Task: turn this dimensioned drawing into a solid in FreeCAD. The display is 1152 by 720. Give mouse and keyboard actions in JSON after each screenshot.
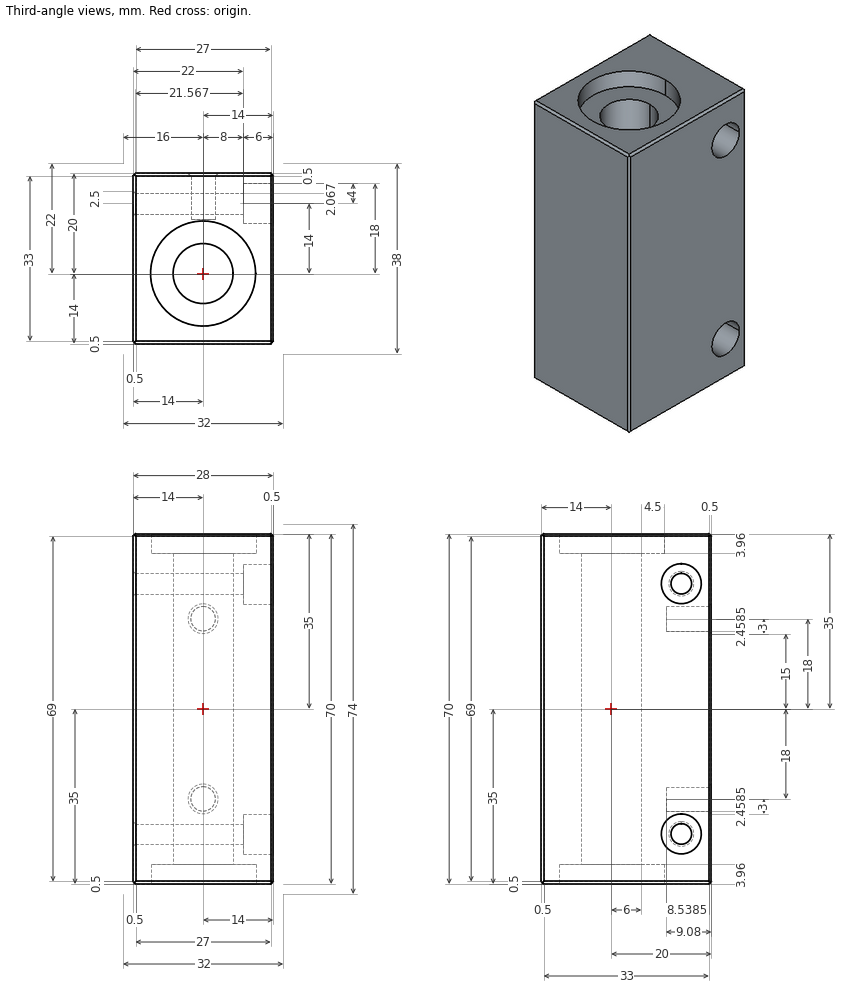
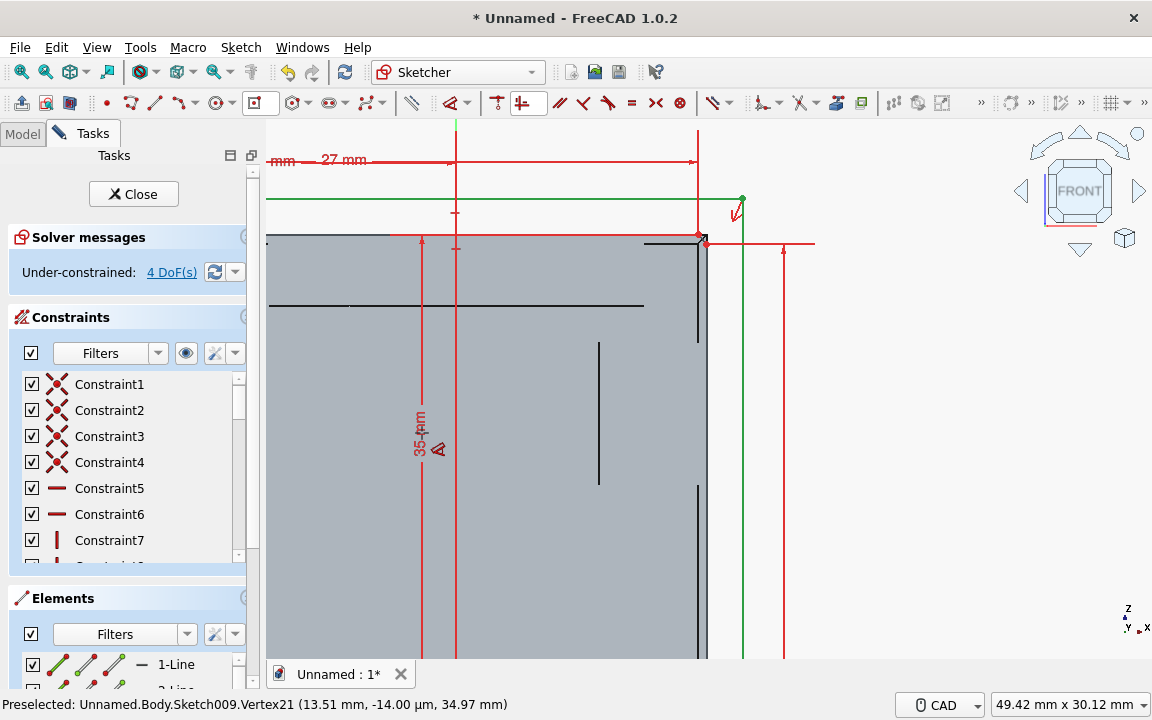
{"action": "scroll", "coordinate": [701, 234], "scroll_direction": "down", "scroll_amount": 7}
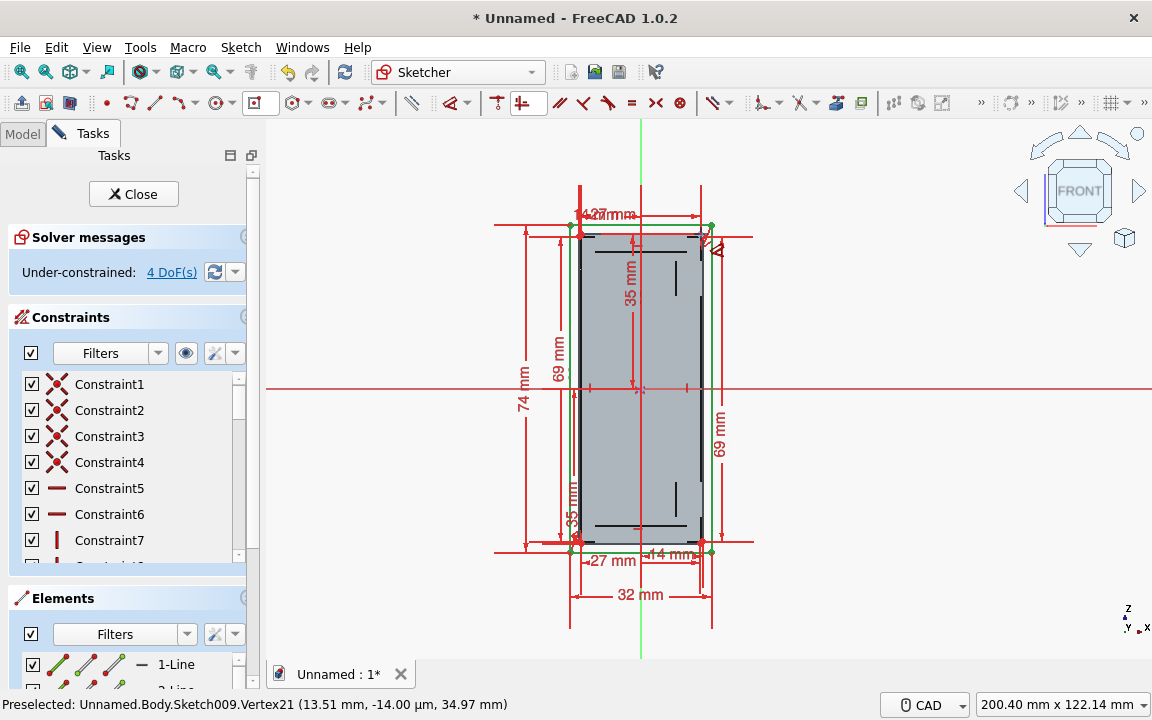
{"action": "scroll", "coordinate": [580, 543], "scroll_direction": "up", "scroll_amount": 15}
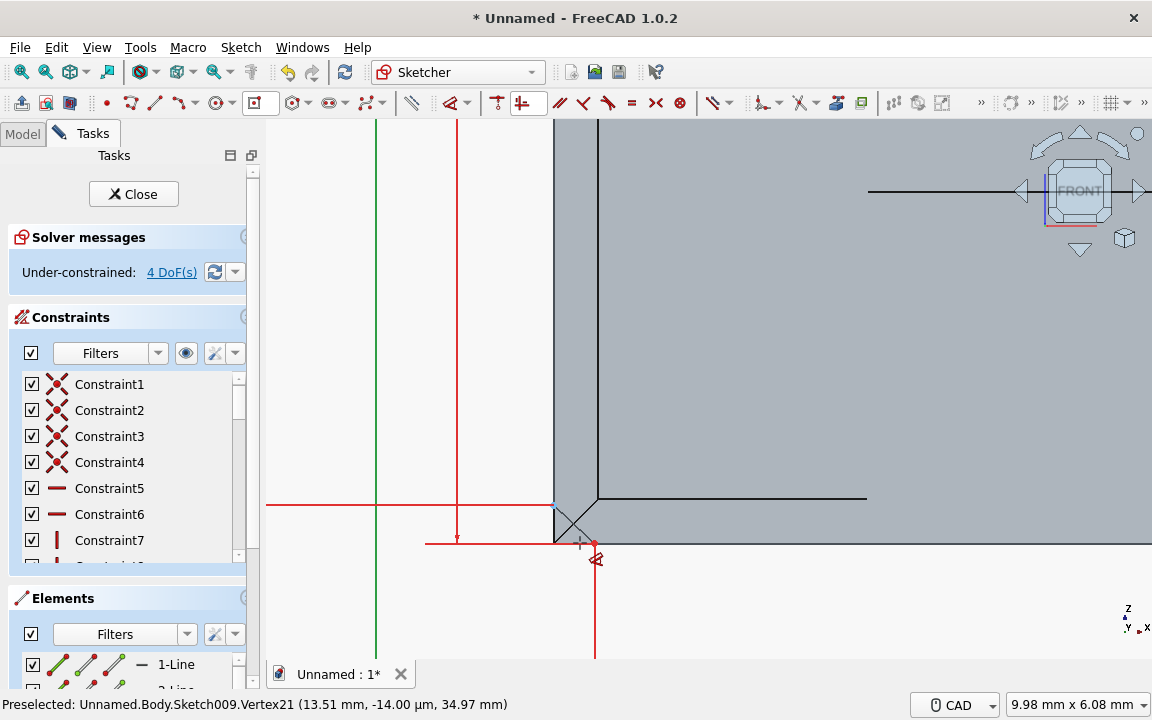
{"action": "left_click", "coordinate": [574, 525]}
{"action": "left_click", "coordinate": [574, 578]}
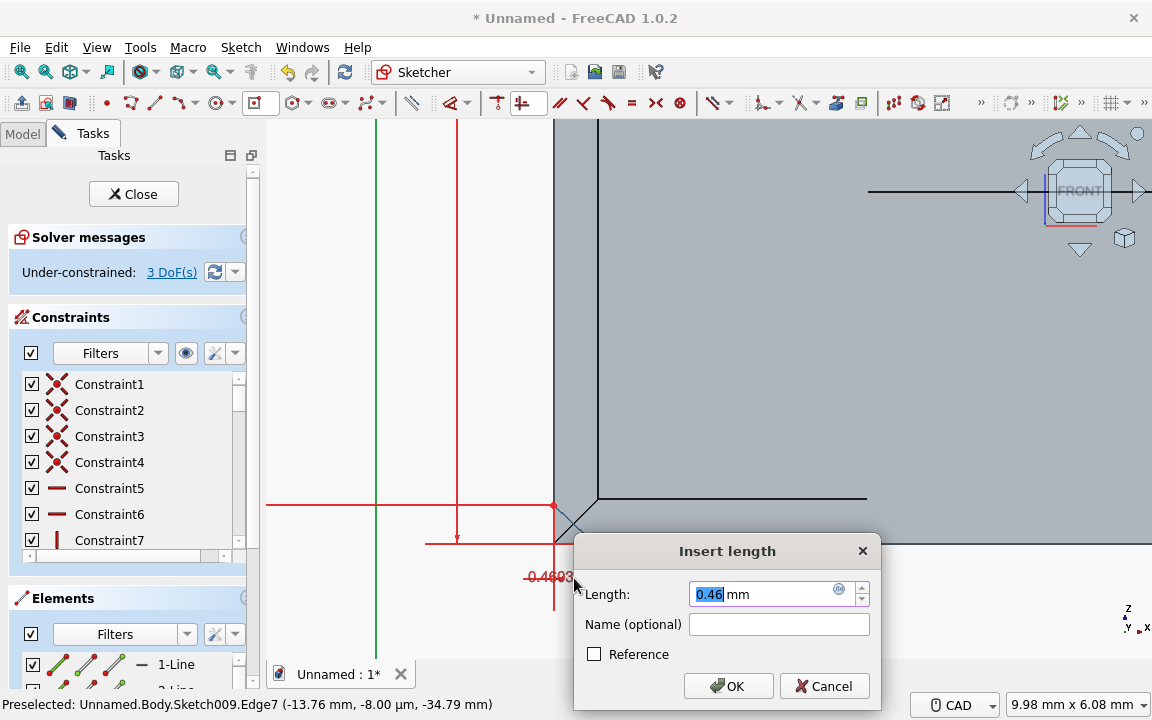
{"action": "type", "text": "0.5"}
{"action": "key", "text": "Return"}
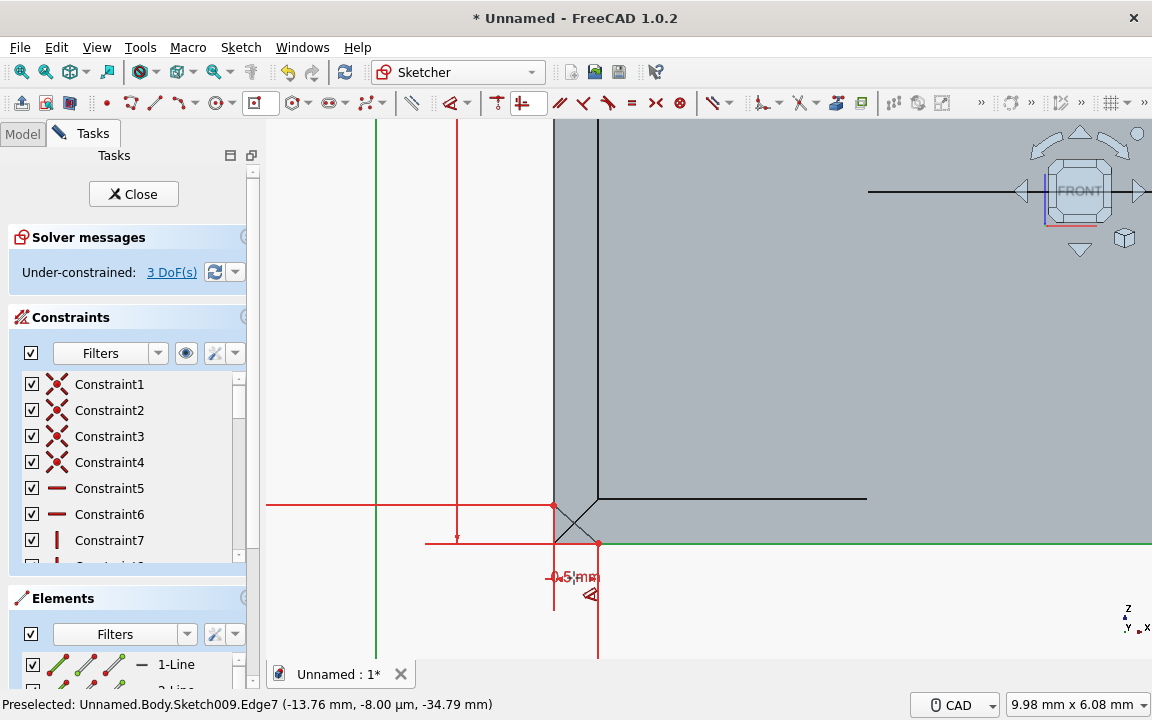
{"action": "left_click", "coordinate": [567, 517]}
{"action": "left_click", "coordinate": [520, 525]}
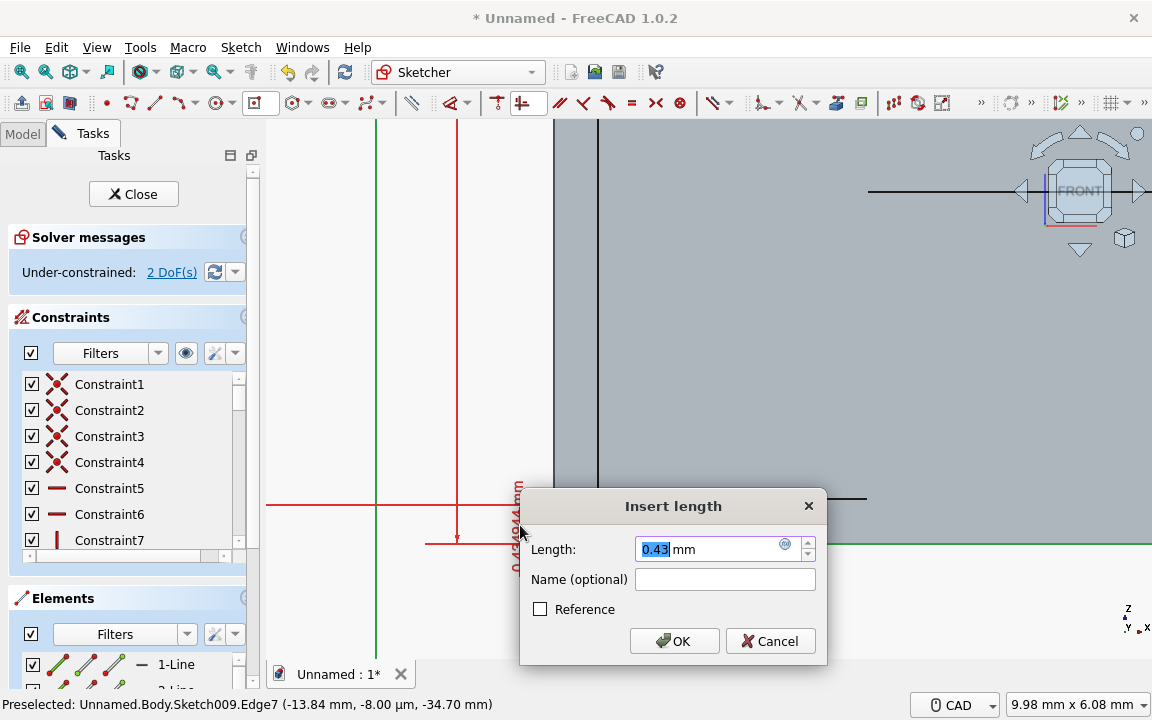
{"action": "type", "text": "0.5"}
{"action": "key", "text": "Return"}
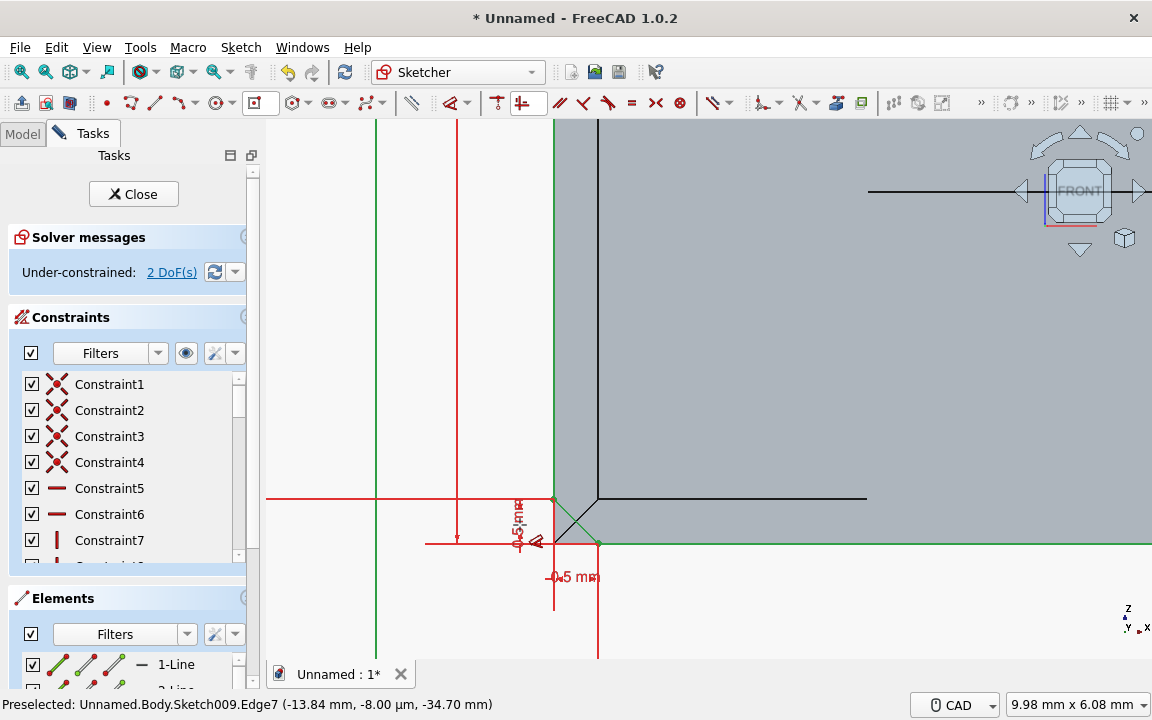
{"action": "scroll", "coordinate": [580, 544], "scroll_direction": "down", "scroll_amount": 15}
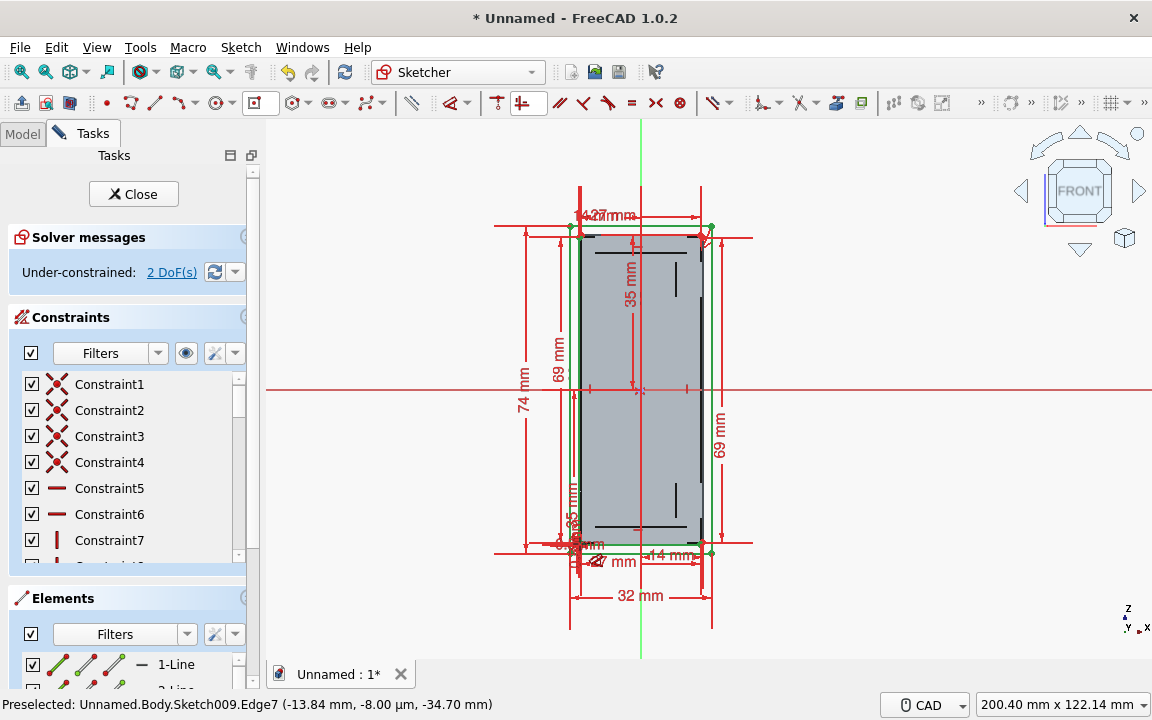
{"action": "scroll", "coordinate": [701, 544], "scroll_direction": "up", "scroll_amount": 15}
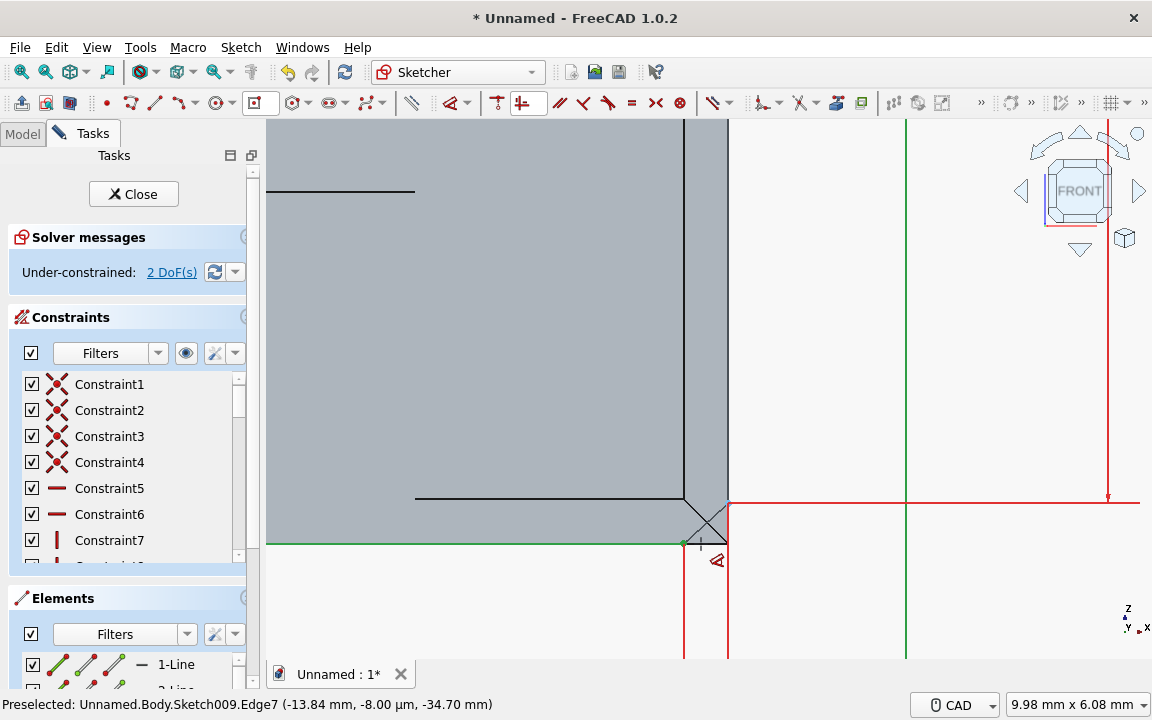
{"action": "left_click", "coordinate": [697, 532]}
{"action": "left_click", "coordinate": [762, 524]}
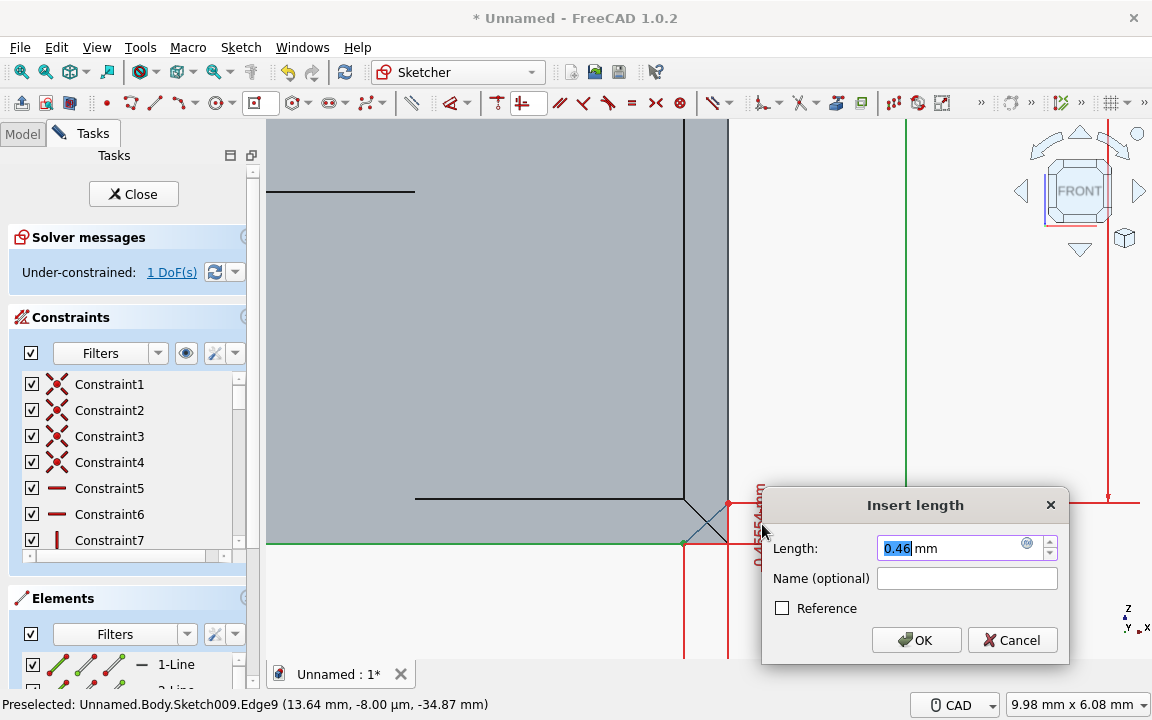
{"action": "type", "text": "0.5"}
{"action": "key", "text": "Return"}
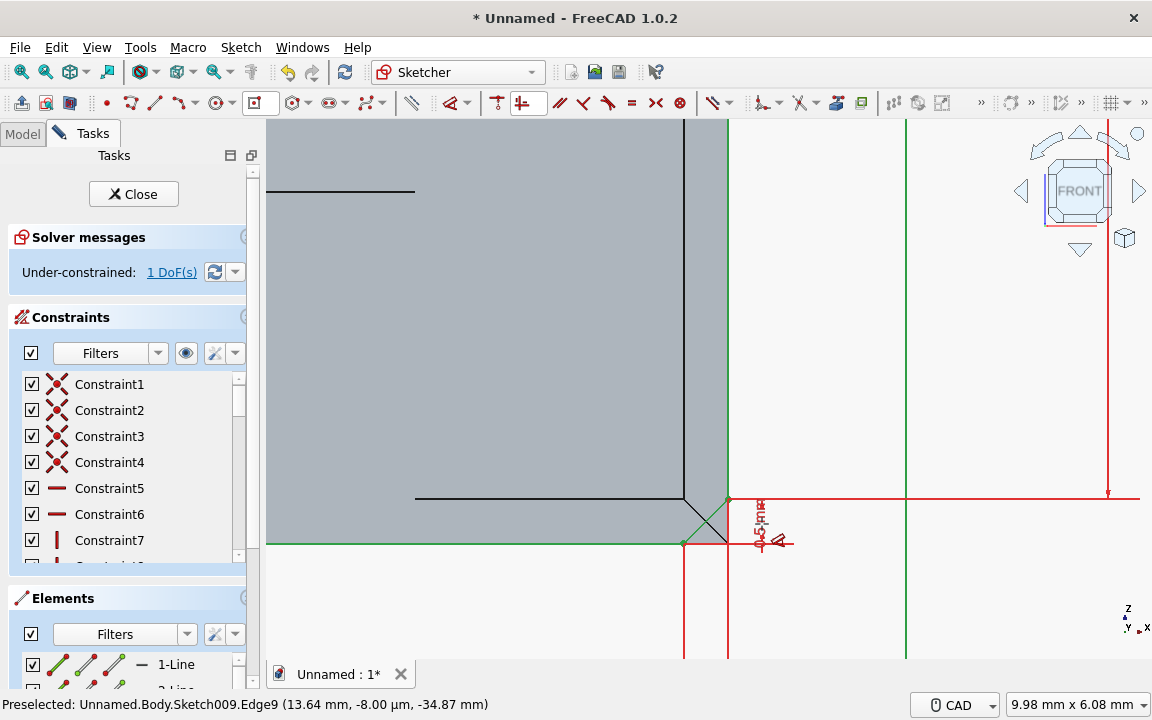
{"action": "scroll", "coordinate": [701, 544], "scroll_direction": "down", "scroll_amount": 15}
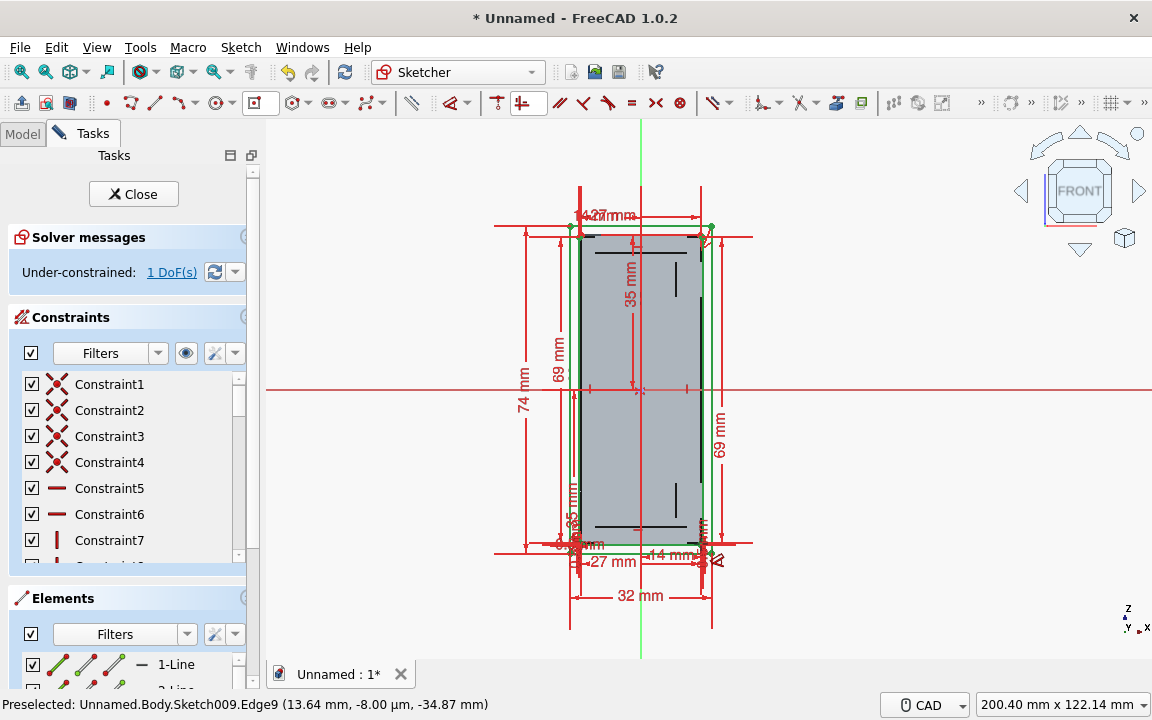
{"action": "scroll", "coordinate": [702, 237], "scroll_direction": "up", "scroll_amount": 15}